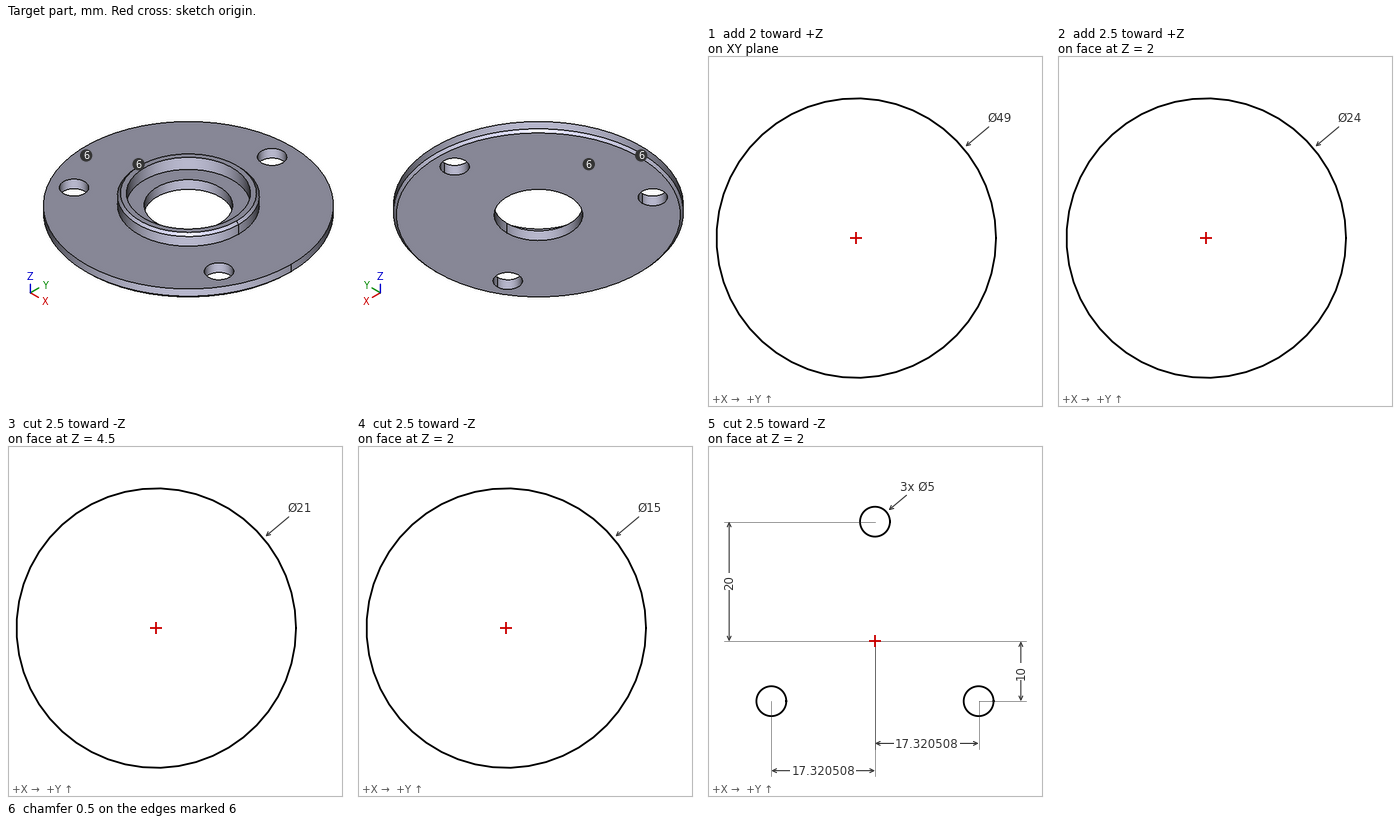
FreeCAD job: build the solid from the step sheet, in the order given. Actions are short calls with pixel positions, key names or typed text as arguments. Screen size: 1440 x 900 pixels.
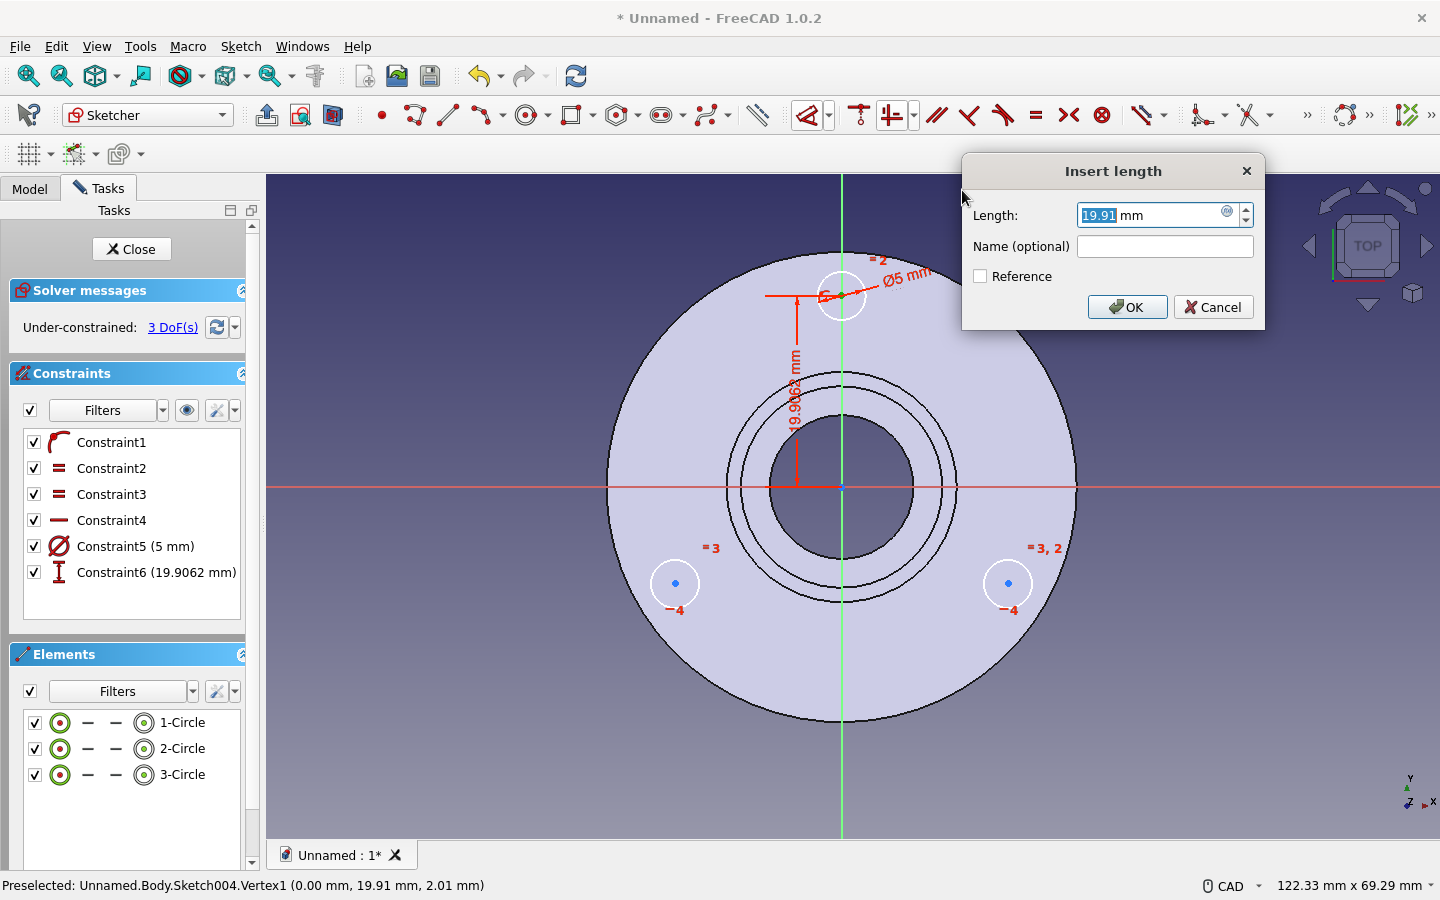
text(20)
key(Return)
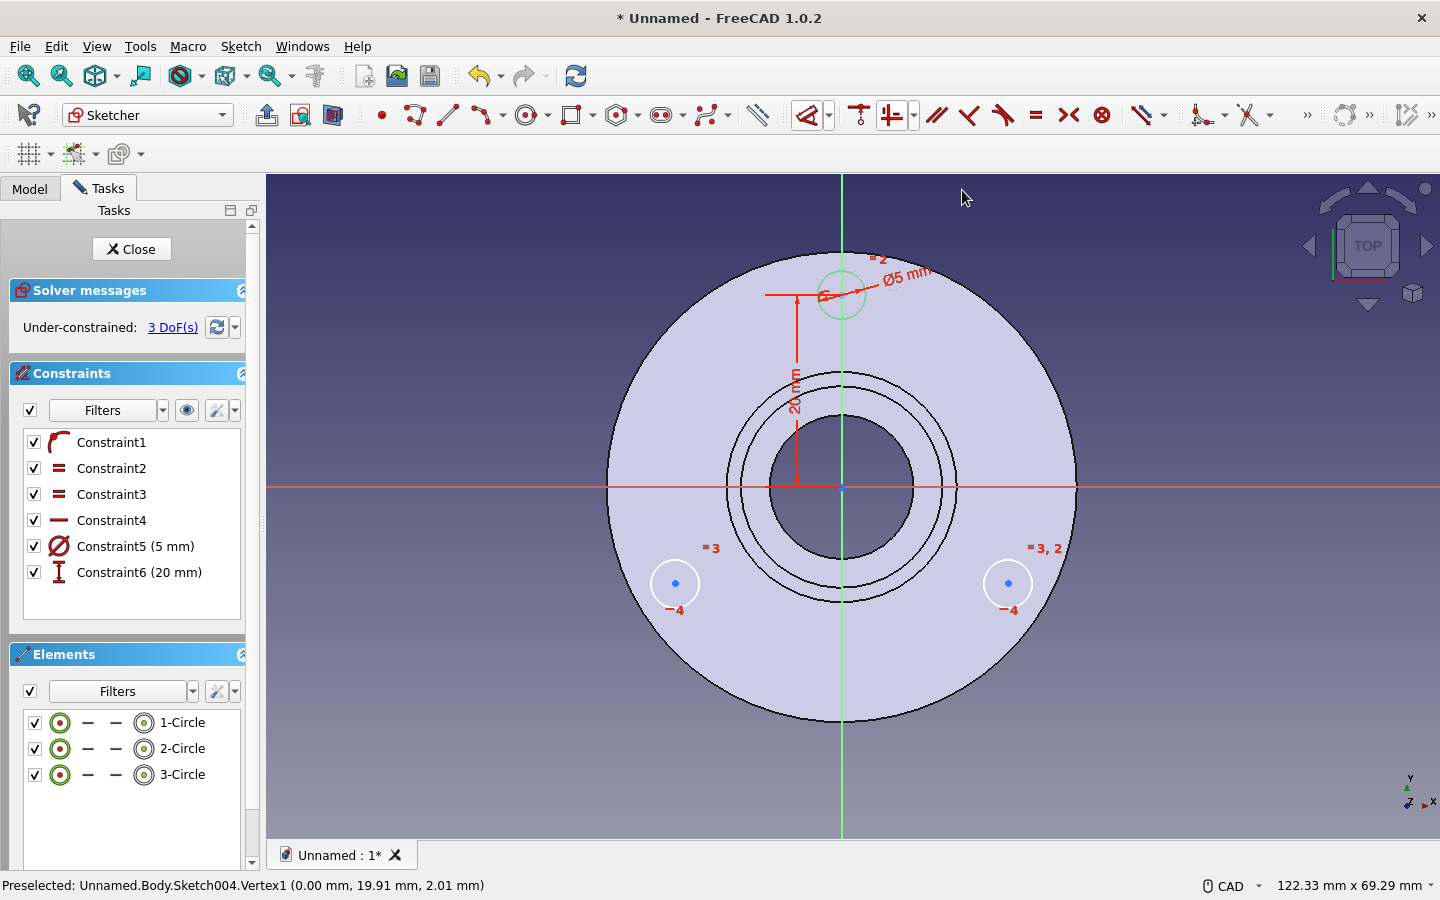
click(1008, 584)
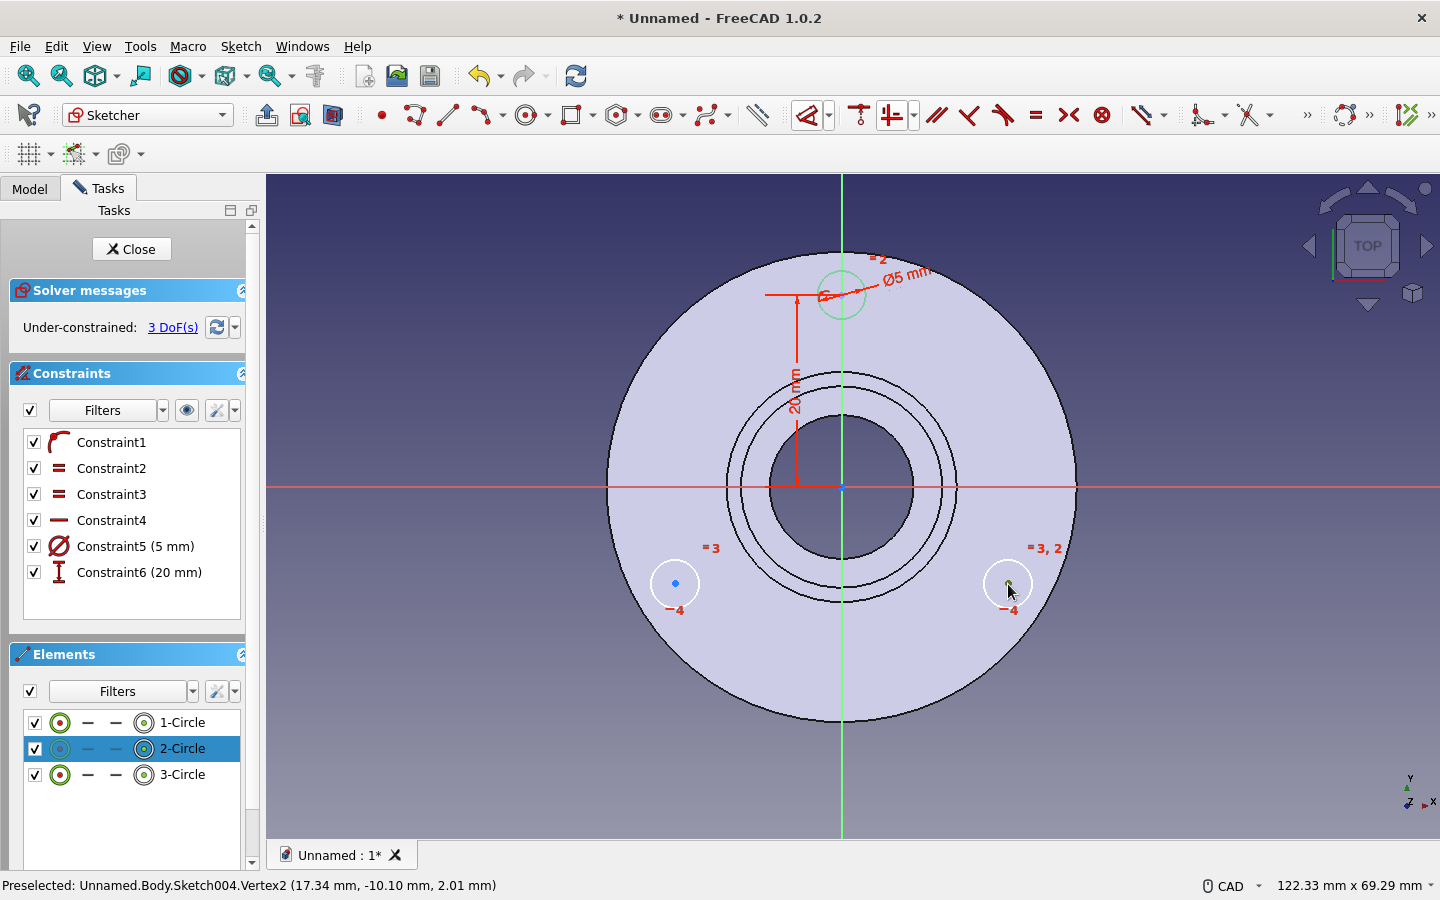
key(i)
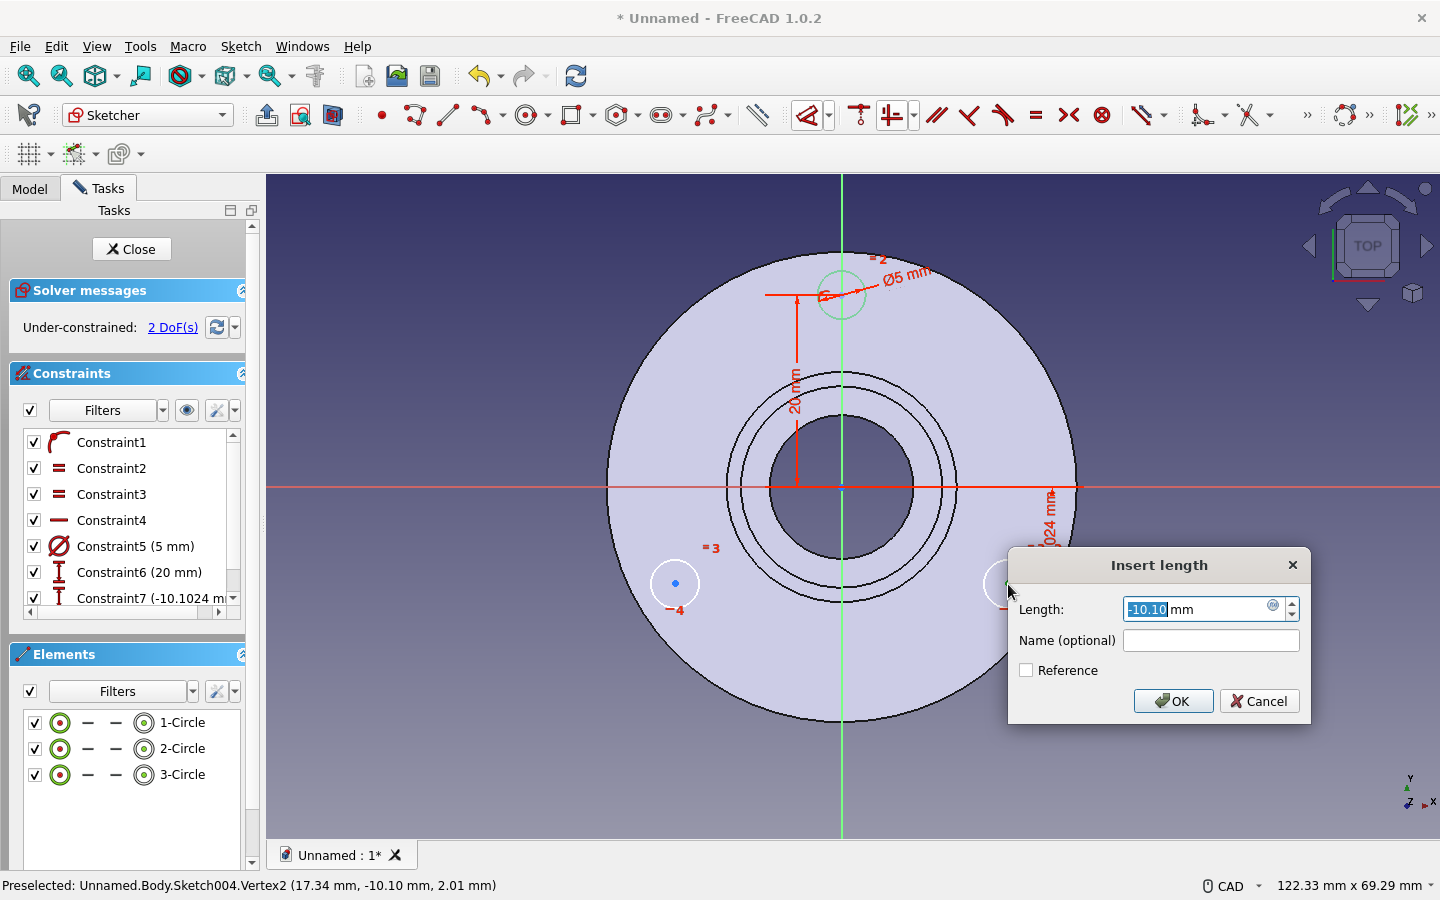
text(-10)
key(Return)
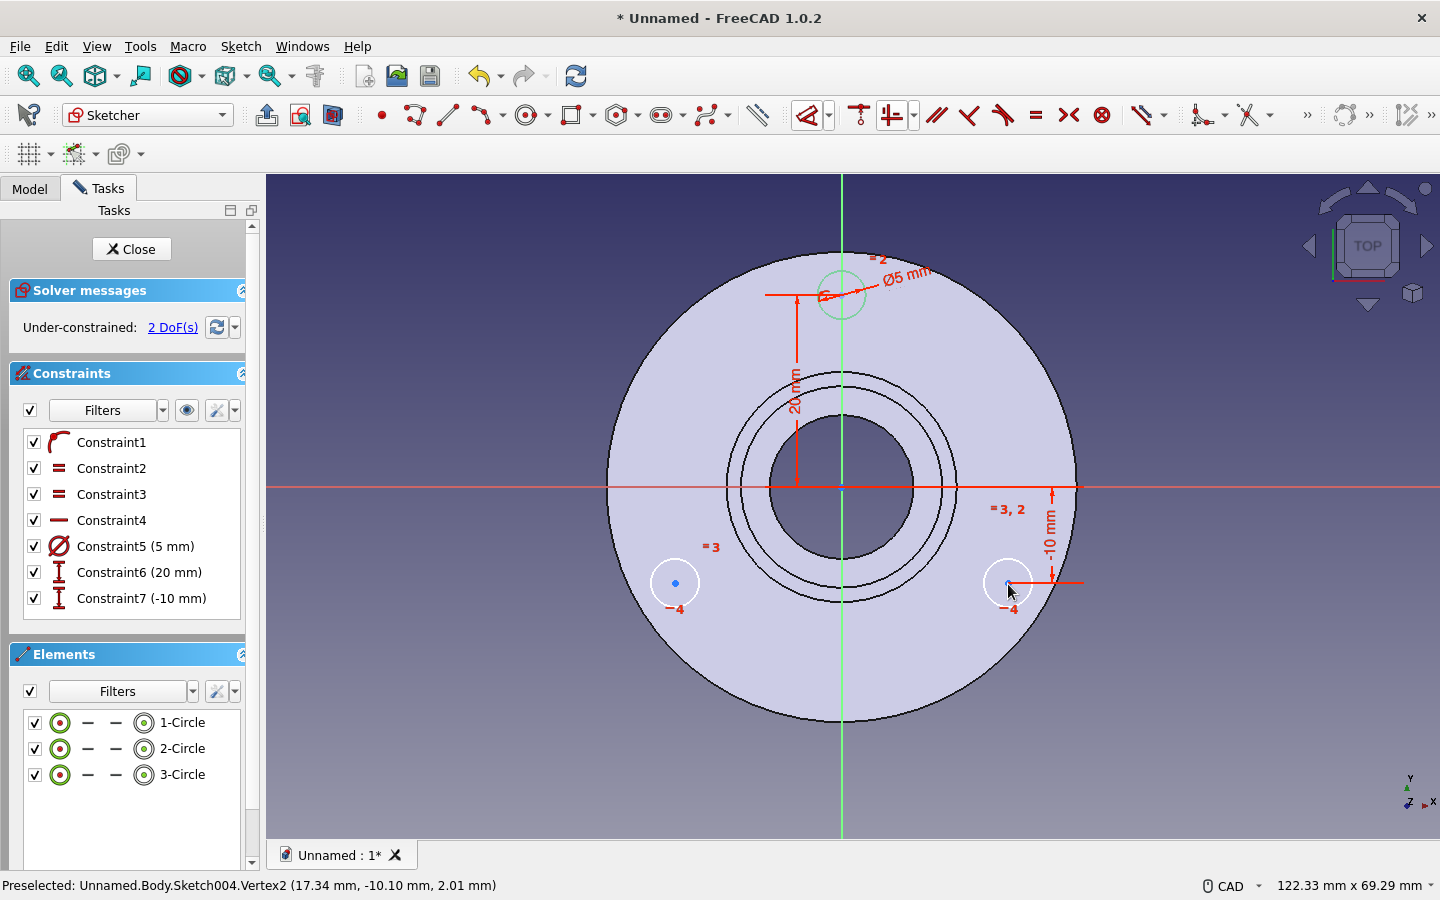
click(1008, 583)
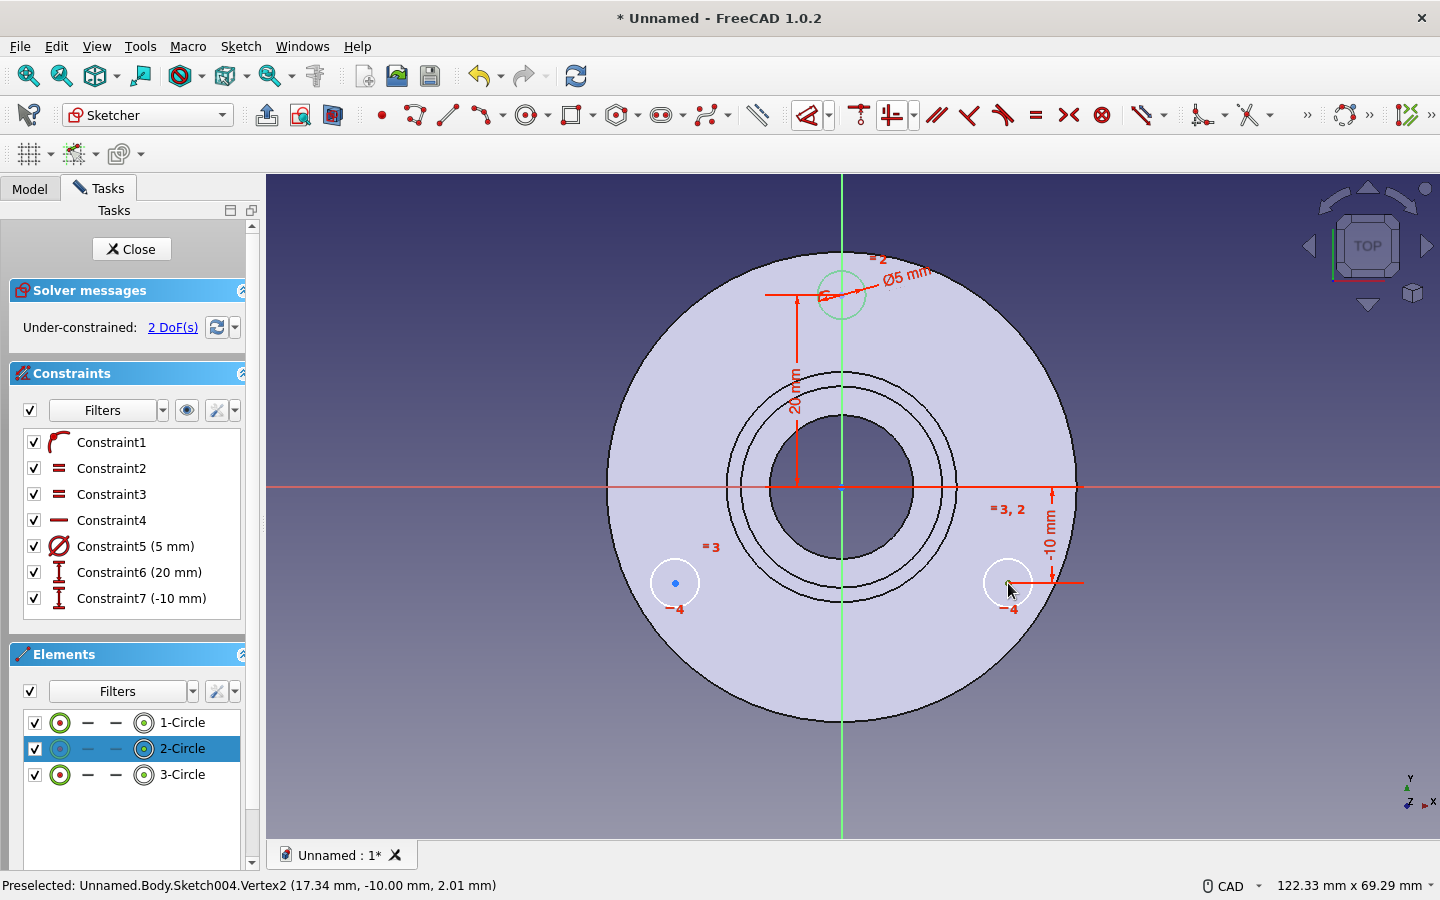
key(l)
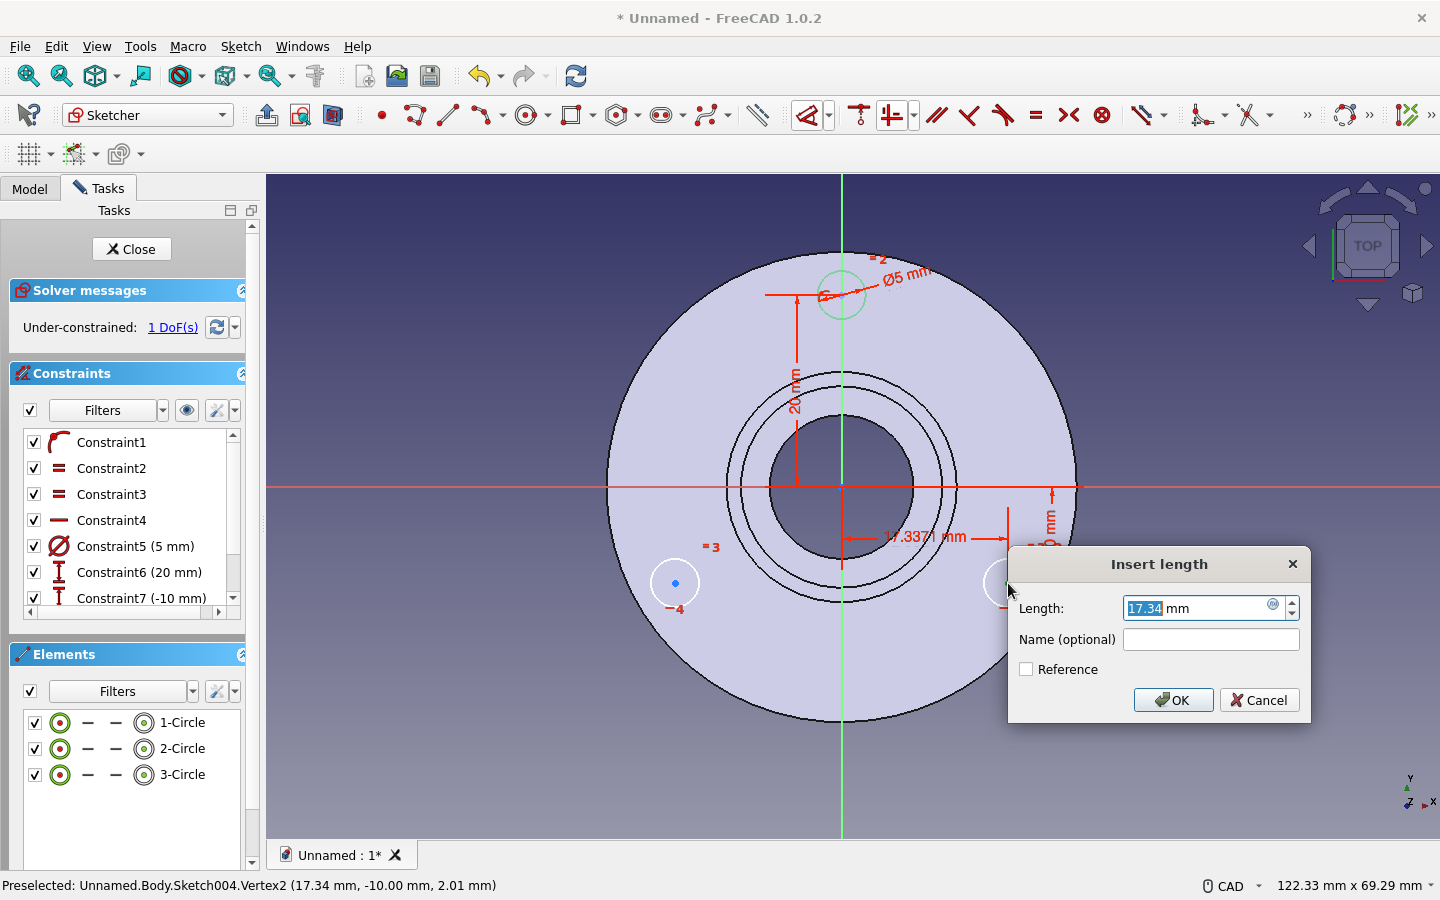
text(17.320508)
key(Return)